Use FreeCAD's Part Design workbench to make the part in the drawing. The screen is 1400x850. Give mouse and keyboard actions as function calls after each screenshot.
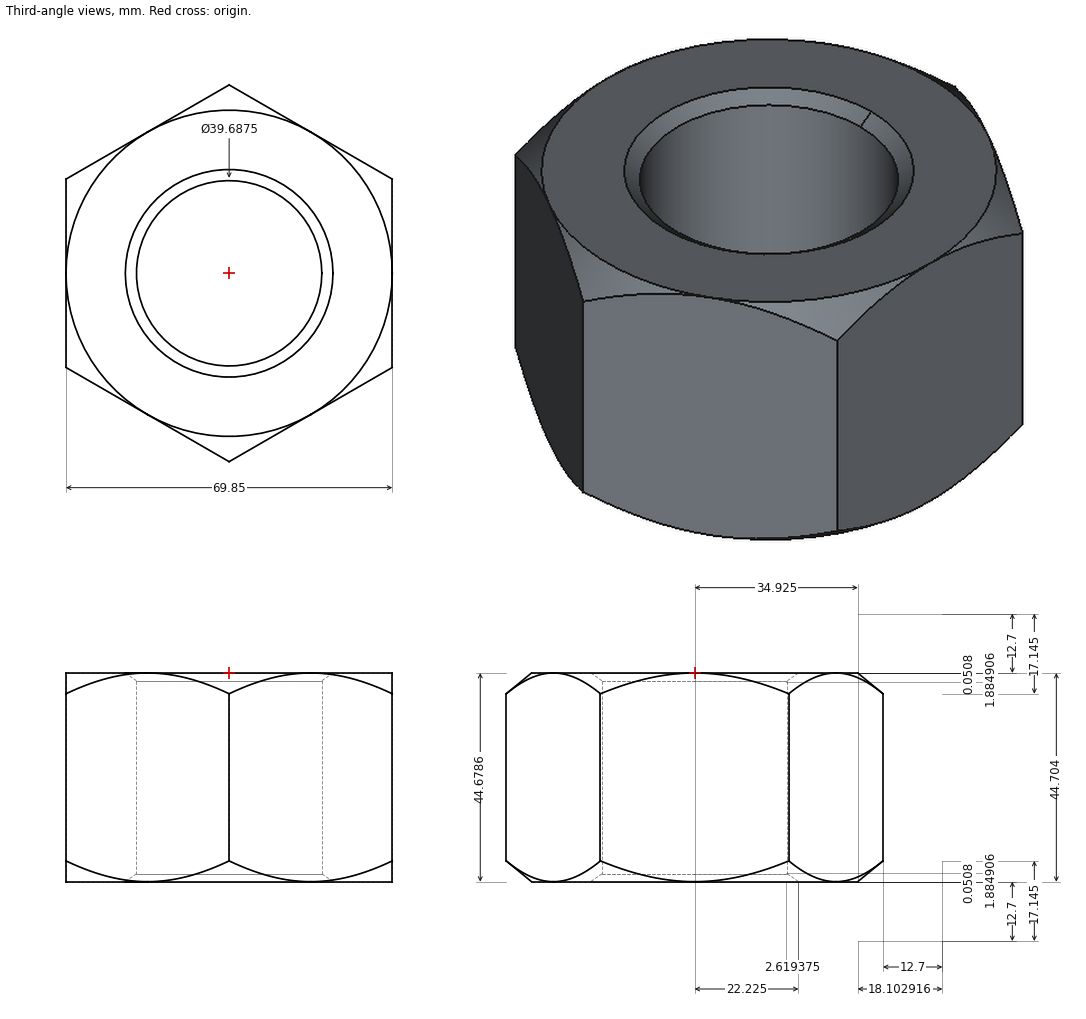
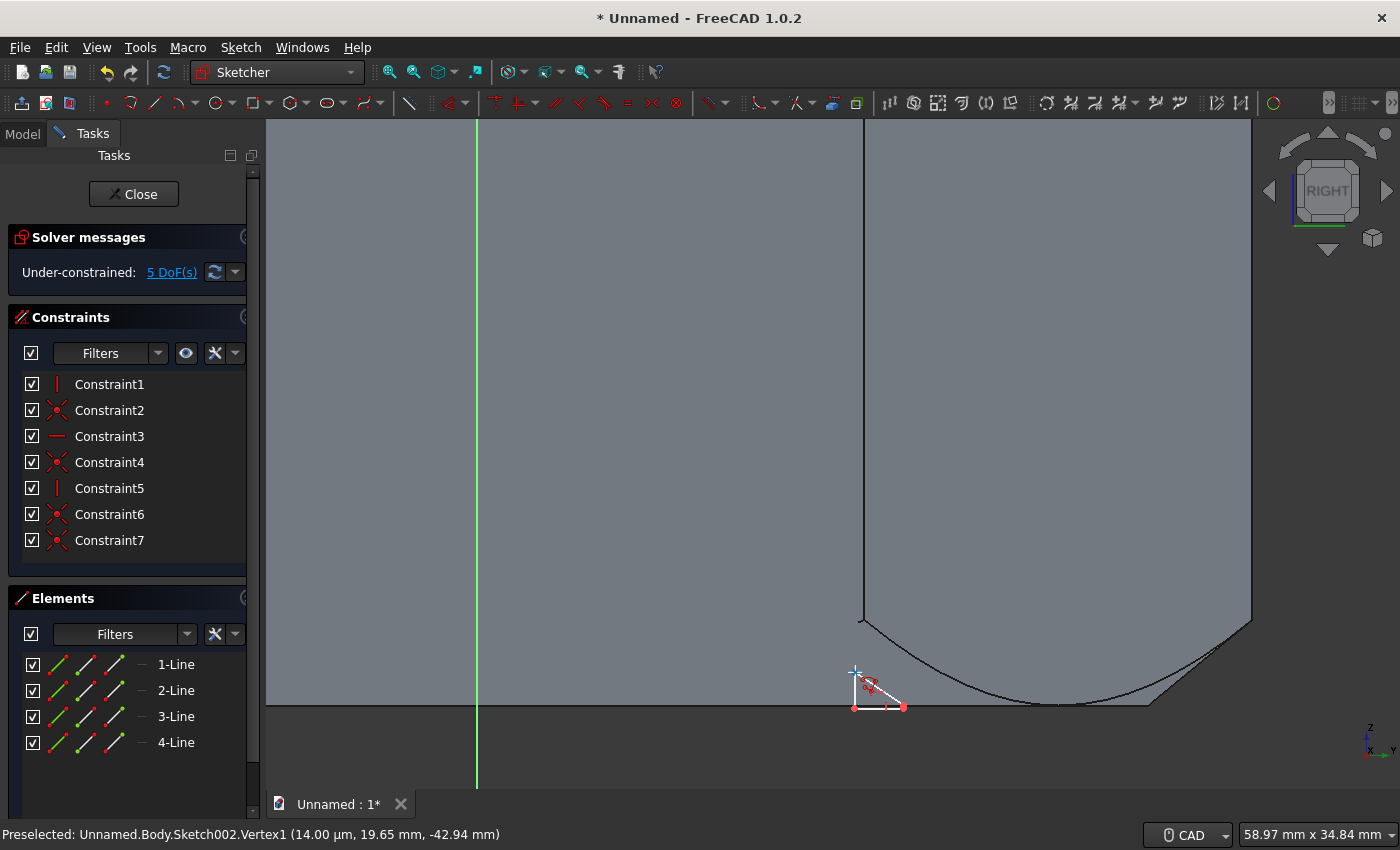
scroll(855, 671, down, 3)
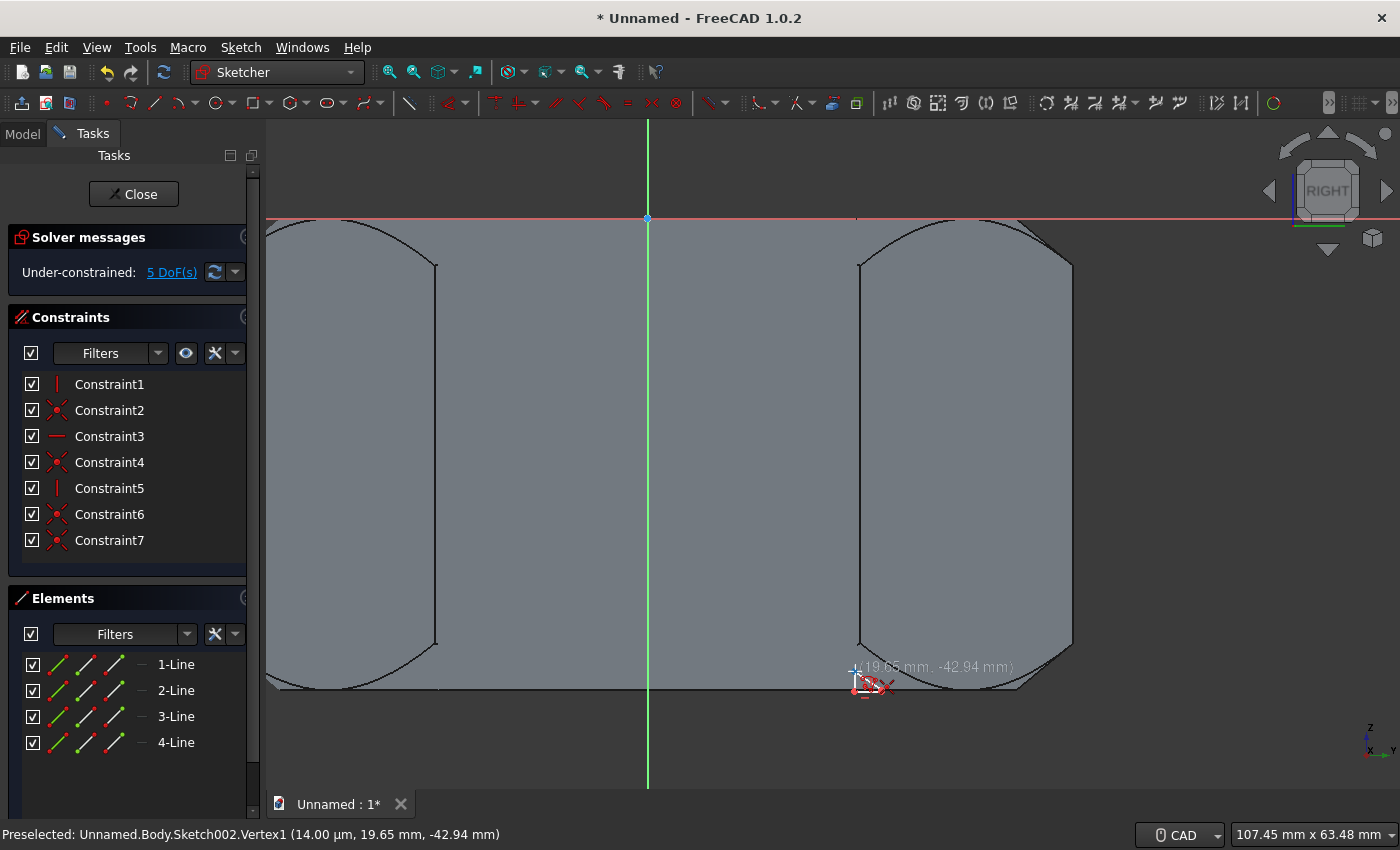
scroll(855, 218, up, 17)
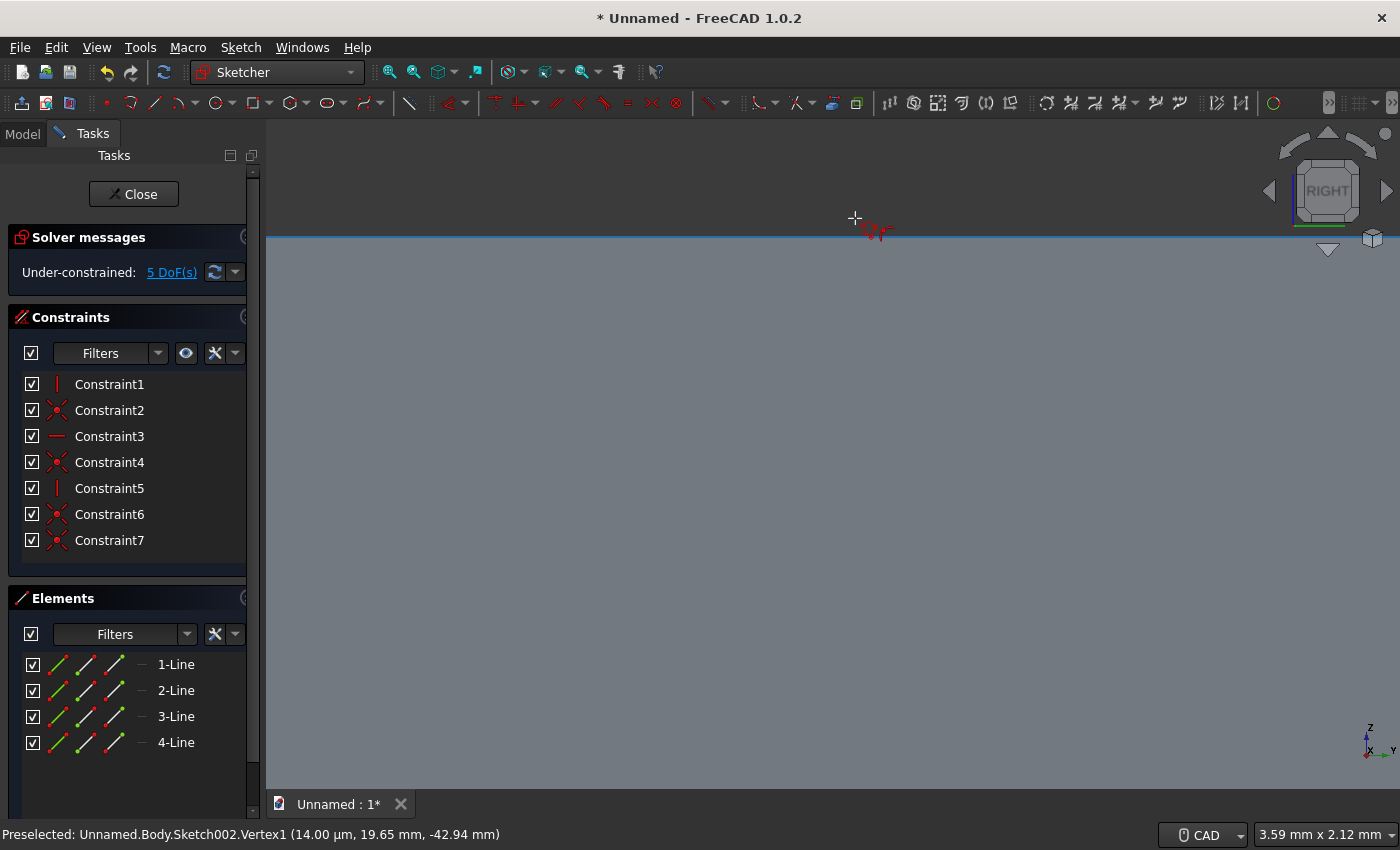
click(825, 221)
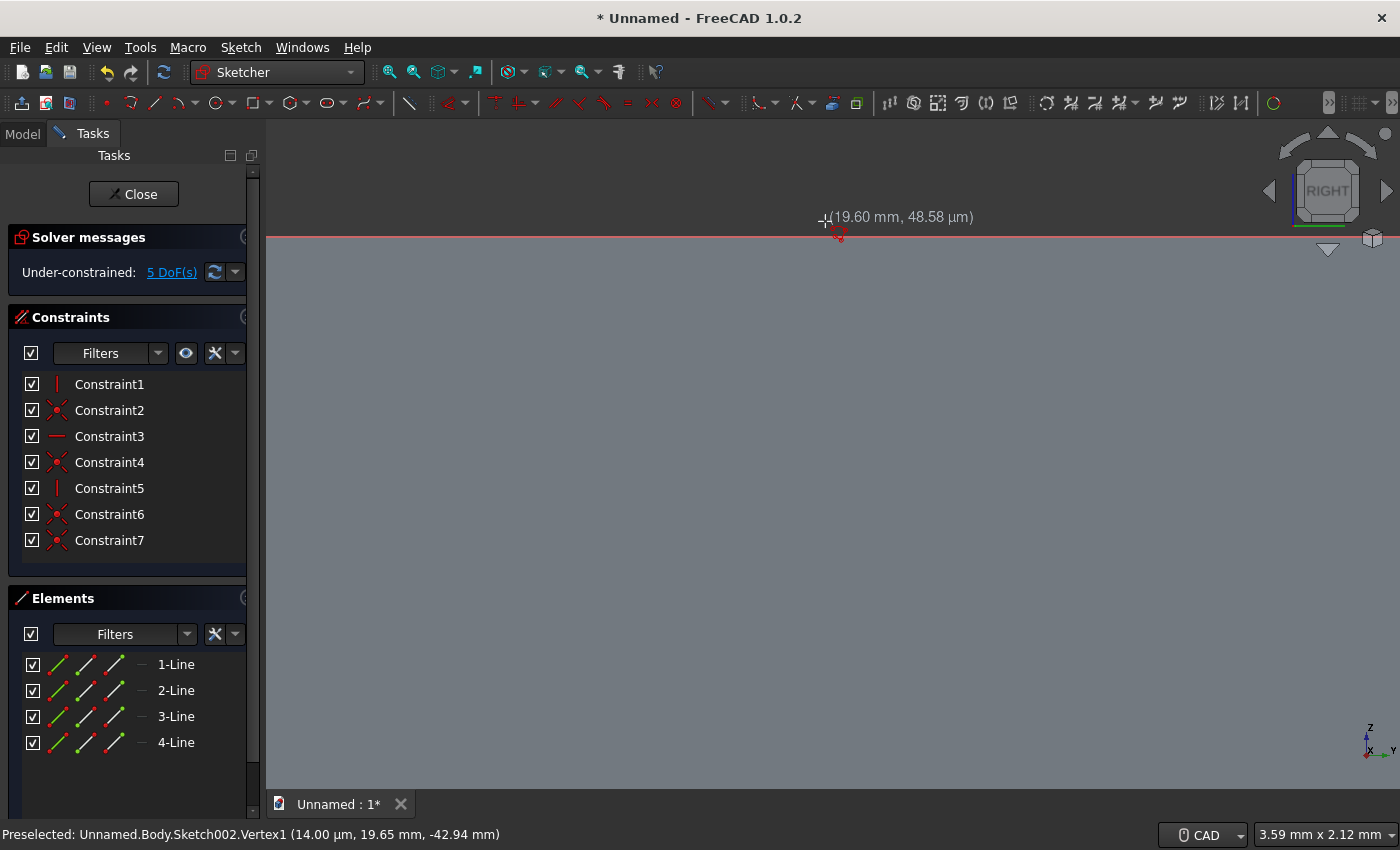
scroll(855, 218, down, 17)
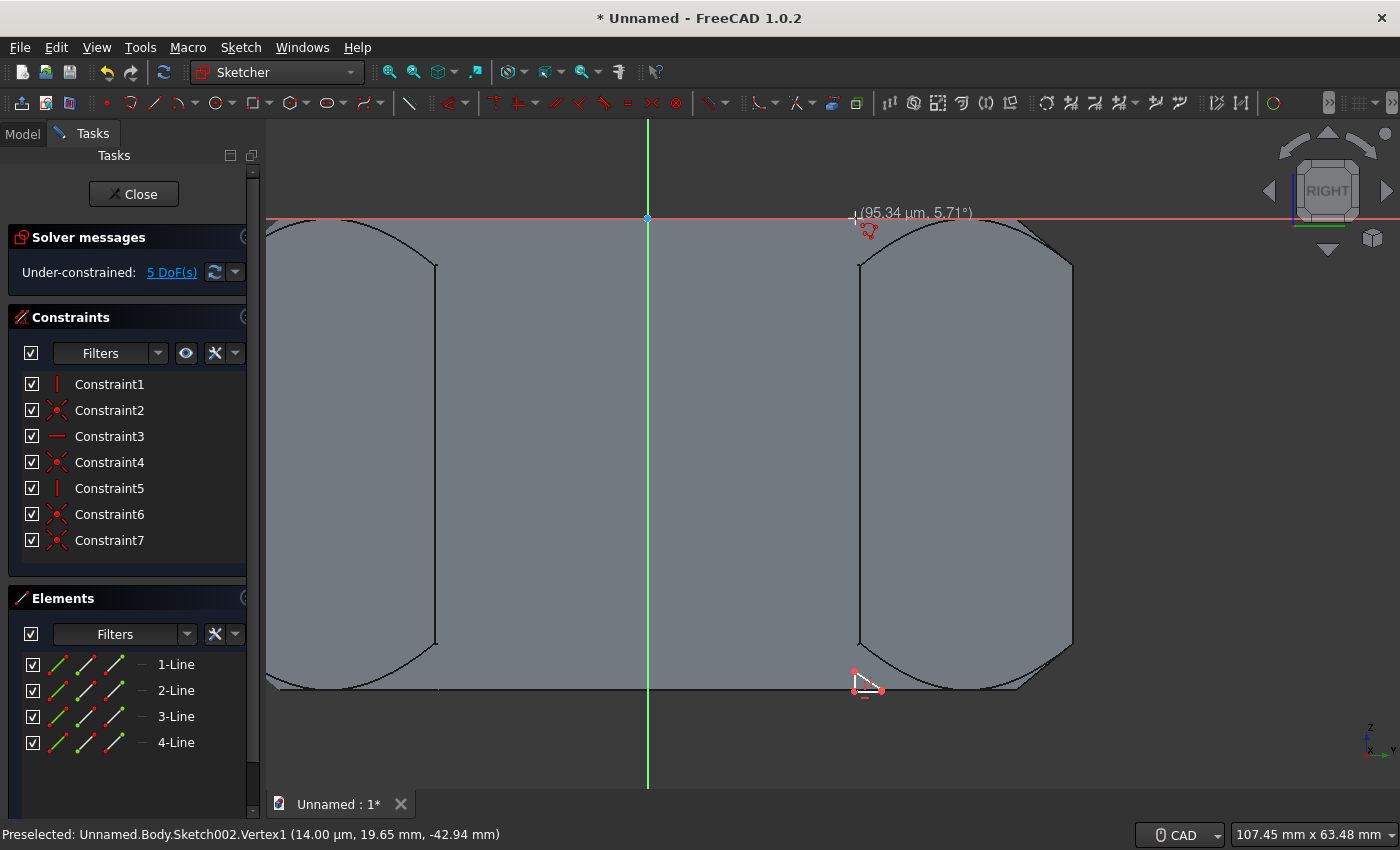
click(855, 238)
click(882, 219)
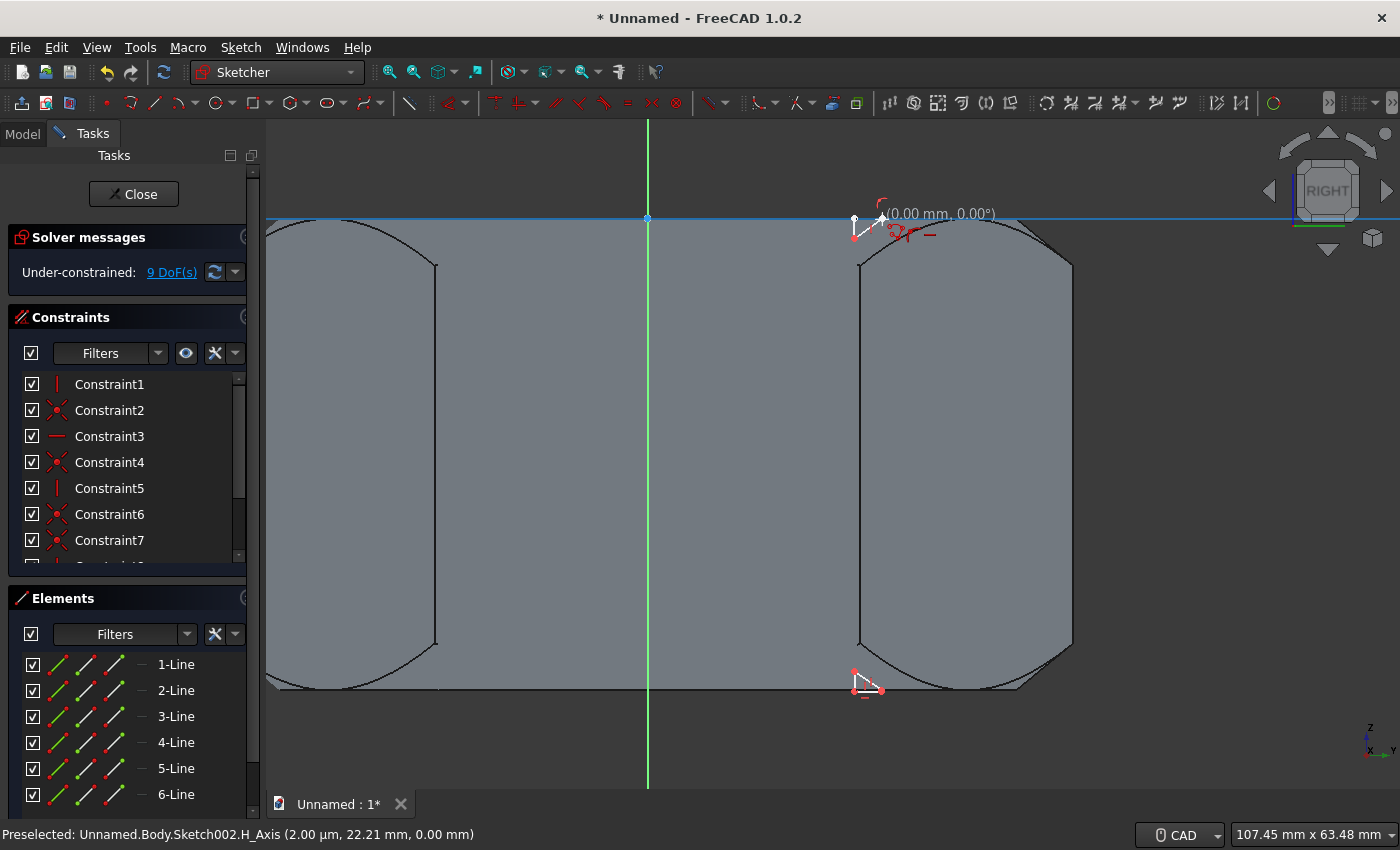
scroll(882, 218, up, 17)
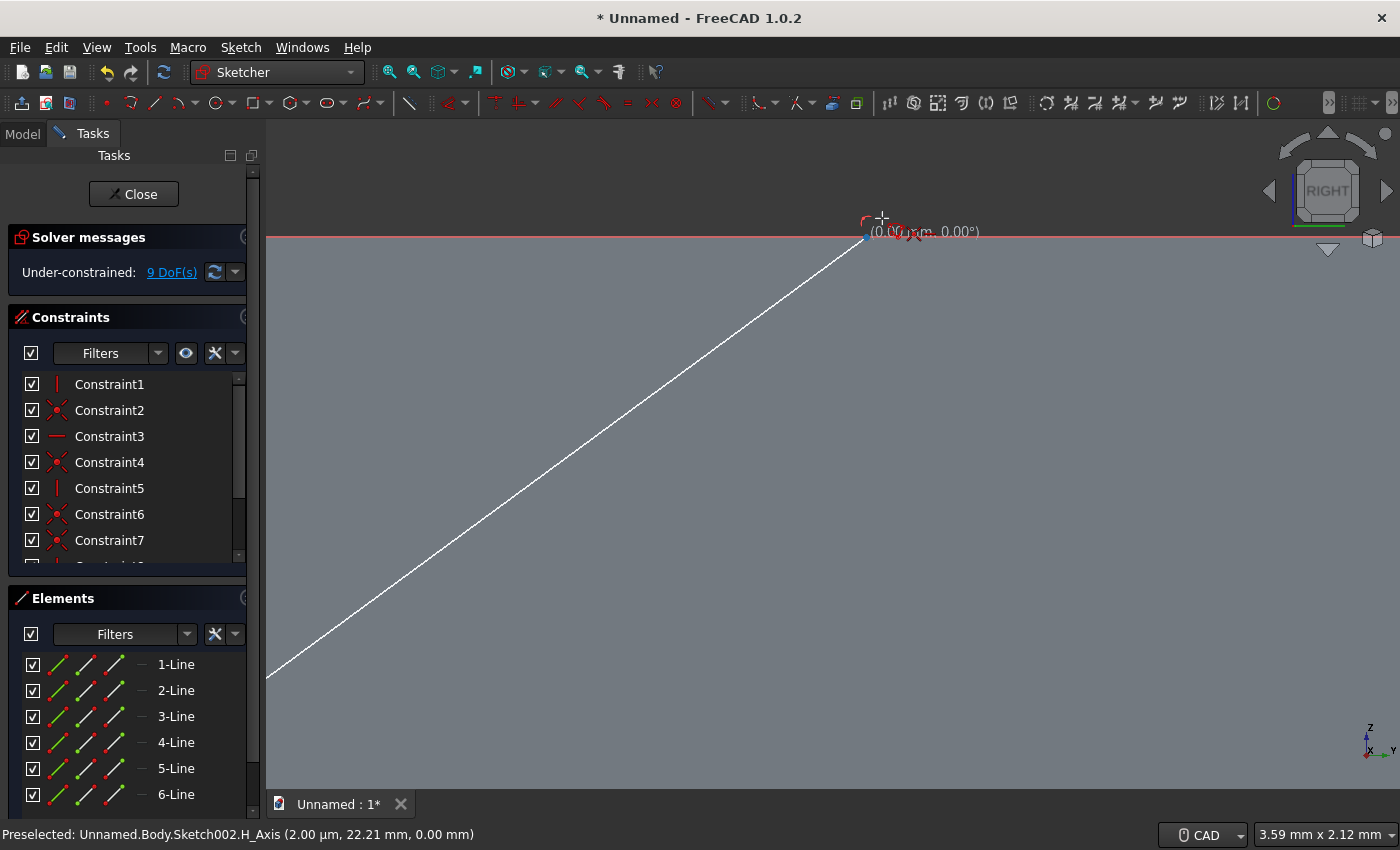
click(866, 221)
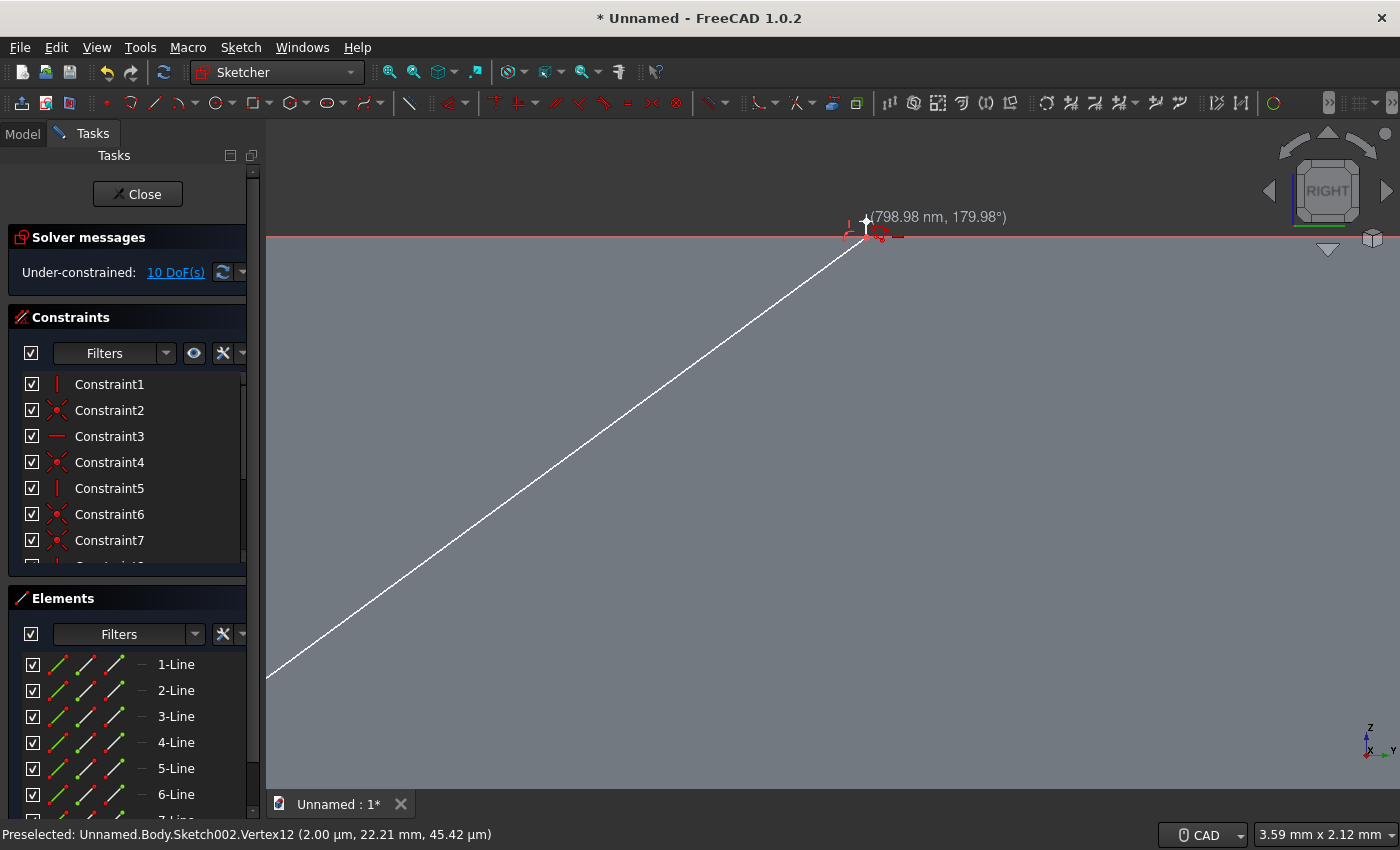
scroll(882, 218, down, 17)